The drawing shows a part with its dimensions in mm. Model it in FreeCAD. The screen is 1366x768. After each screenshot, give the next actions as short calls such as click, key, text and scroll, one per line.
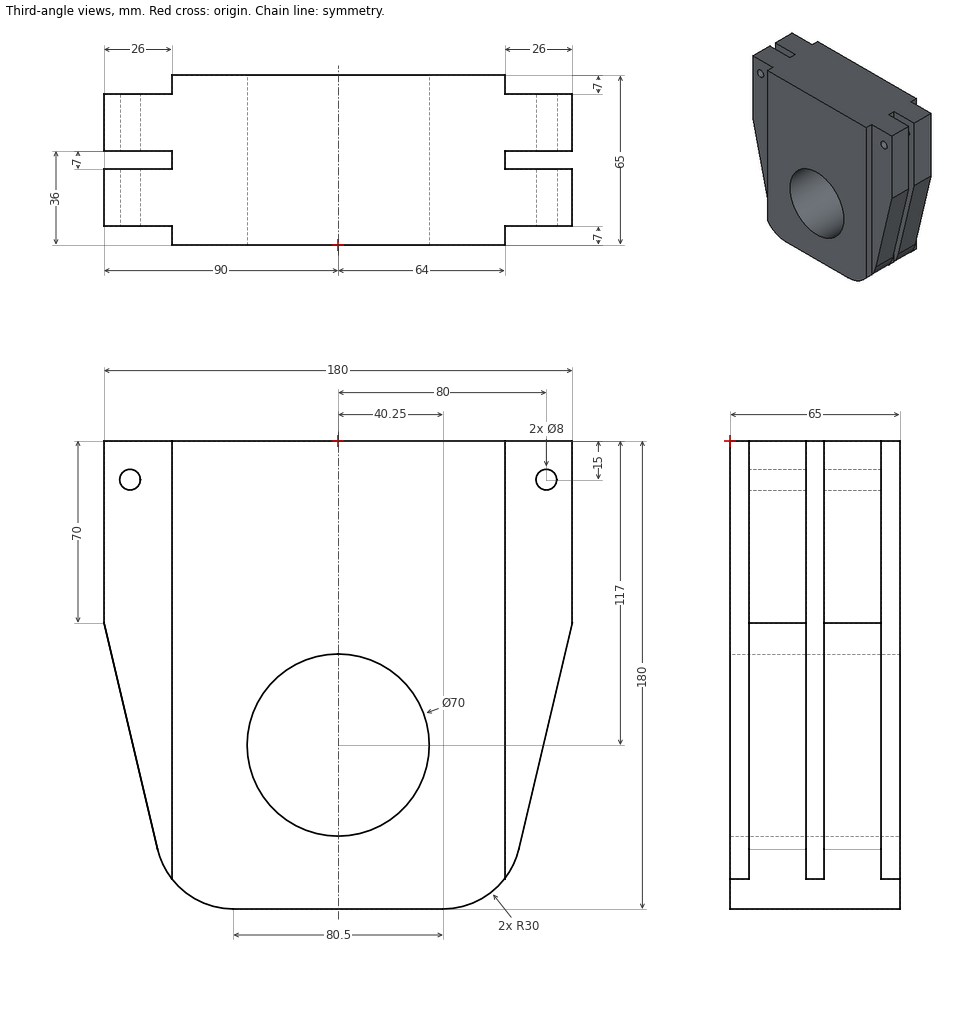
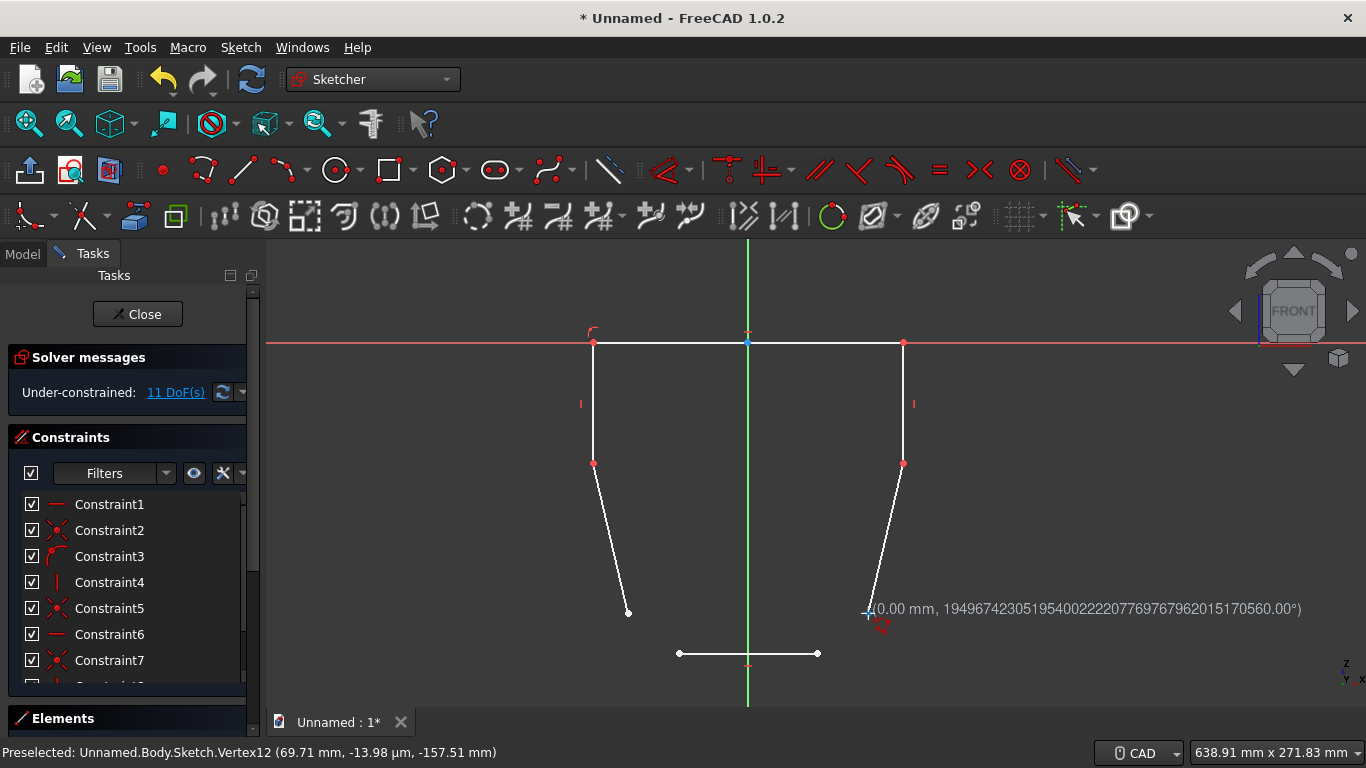
click(284, 170)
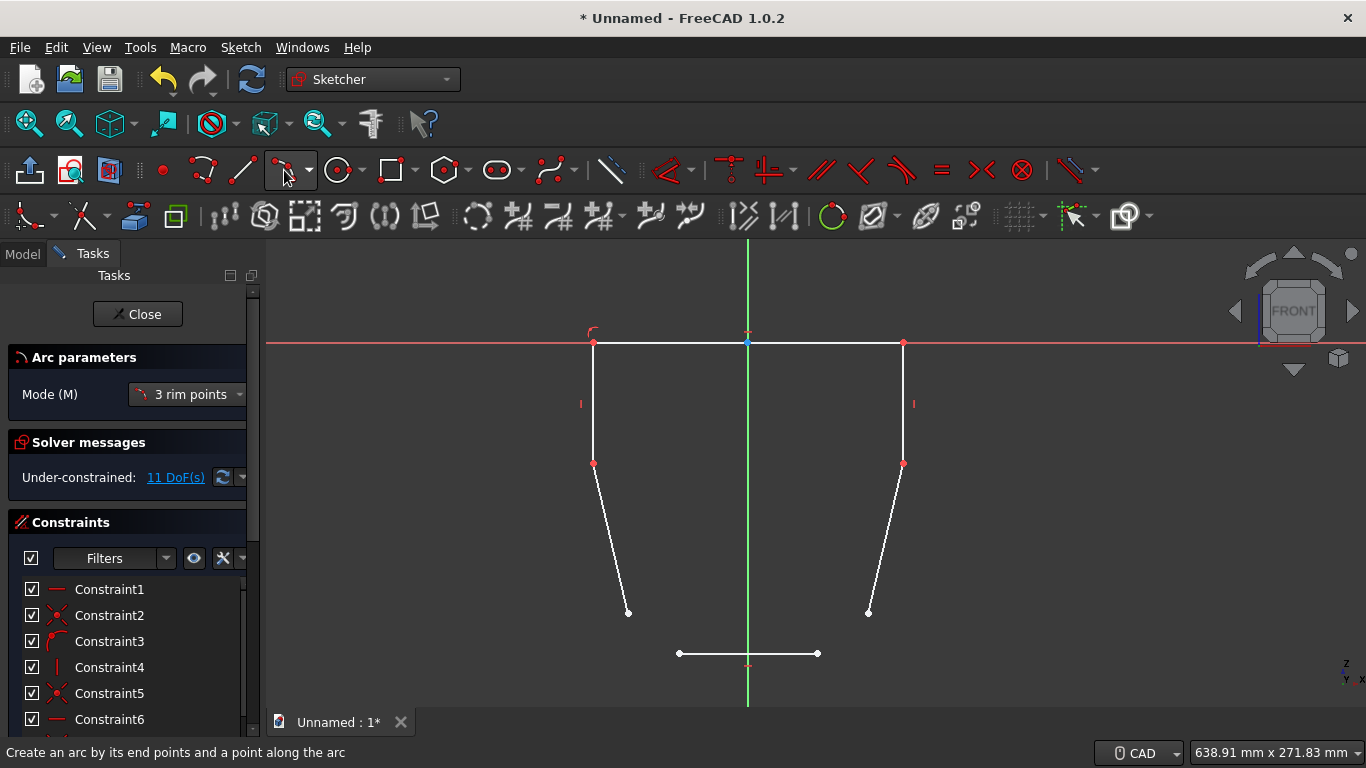
click(679, 654)
click(628, 614)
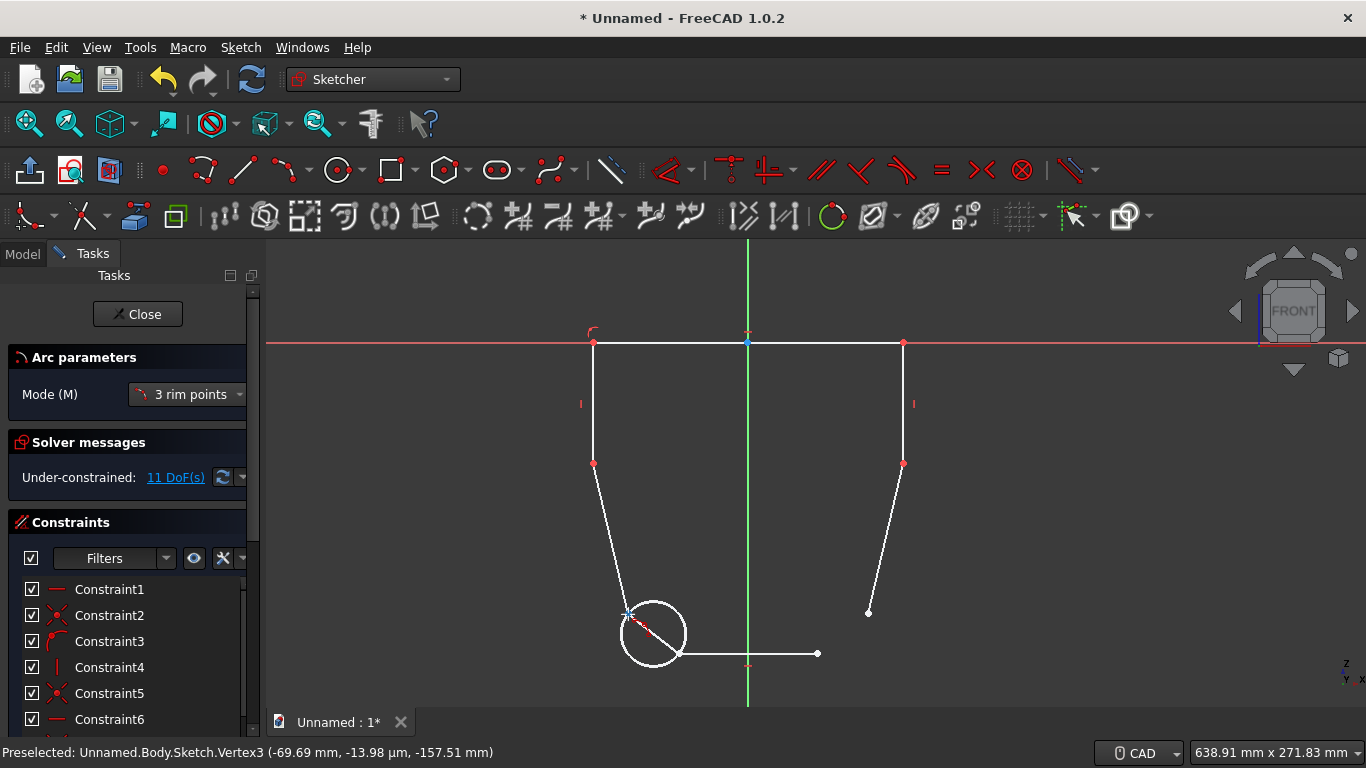
scroll(647, 642, up, 2)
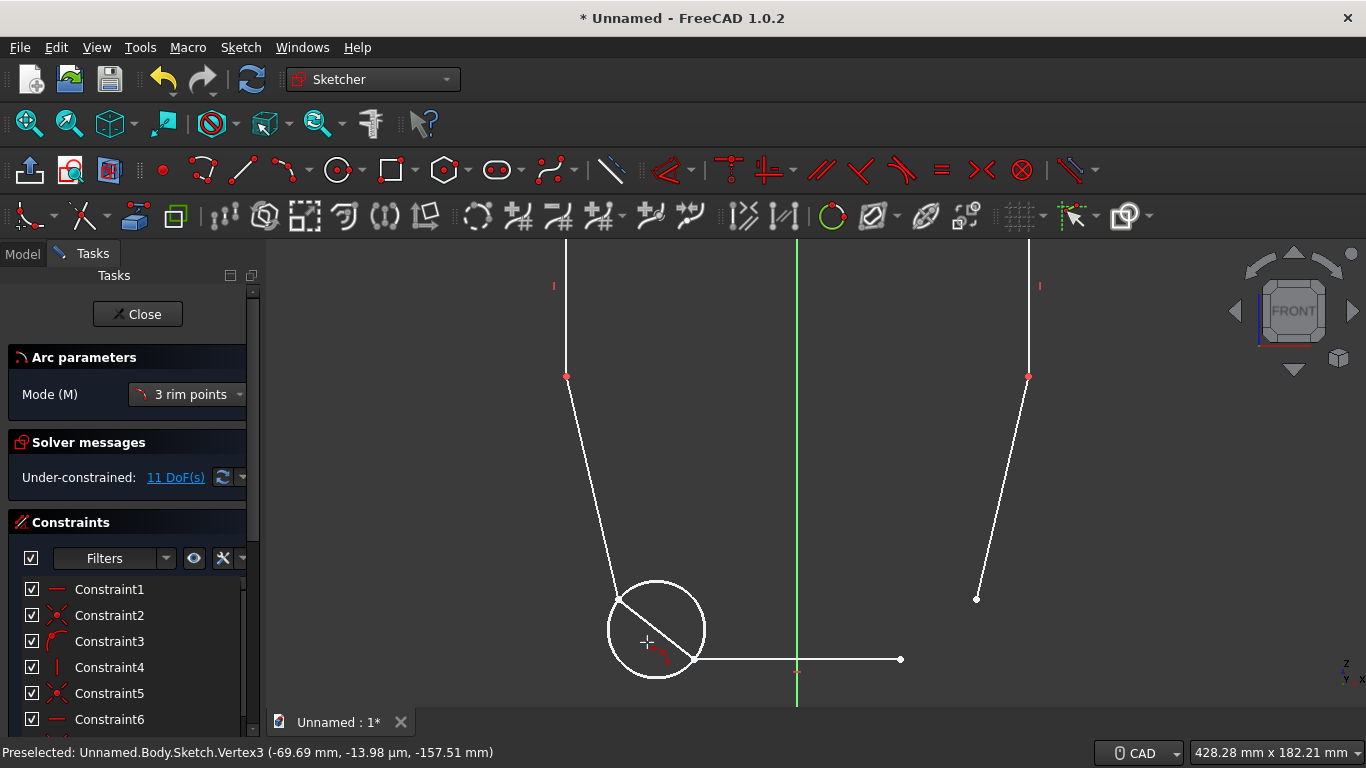
click(646, 641)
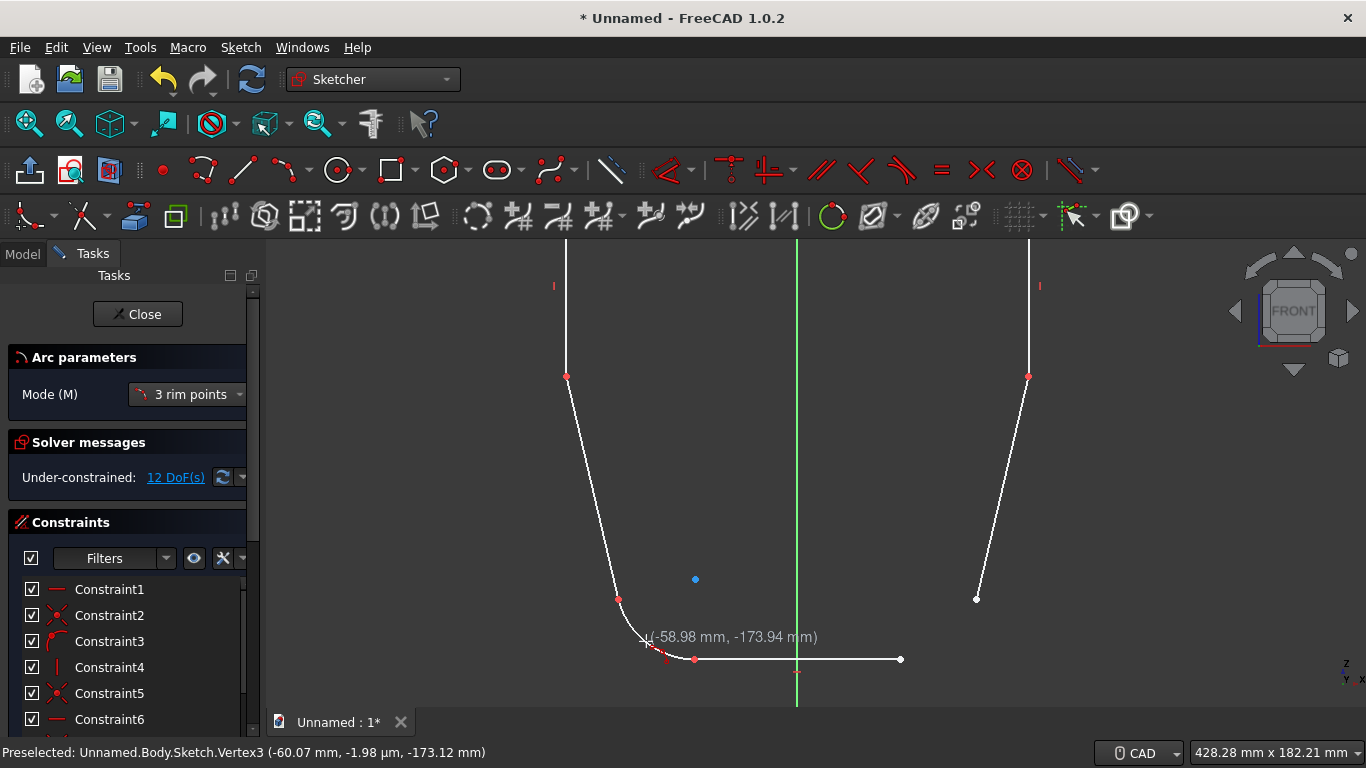
click(977, 600)
click(900, 659)
click(949, 641)
key(Escape)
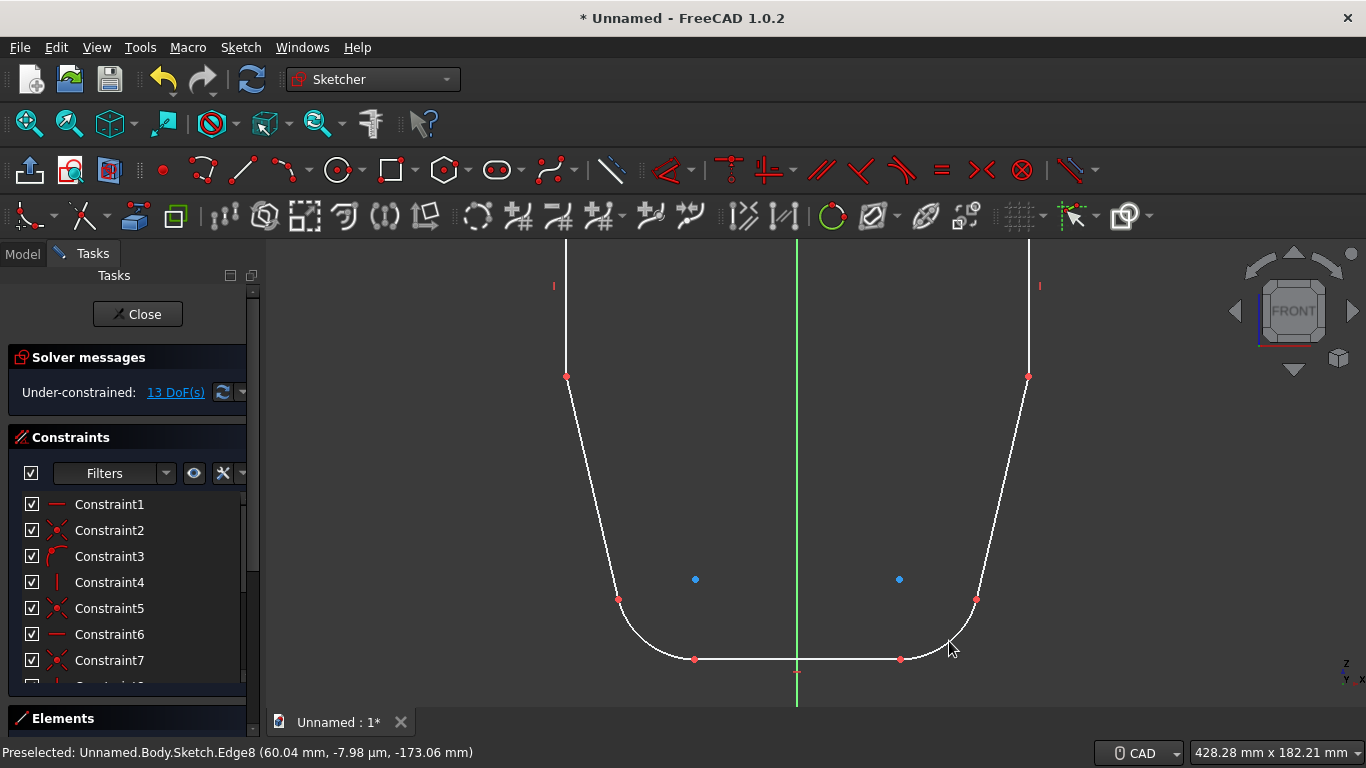
click(839, 659)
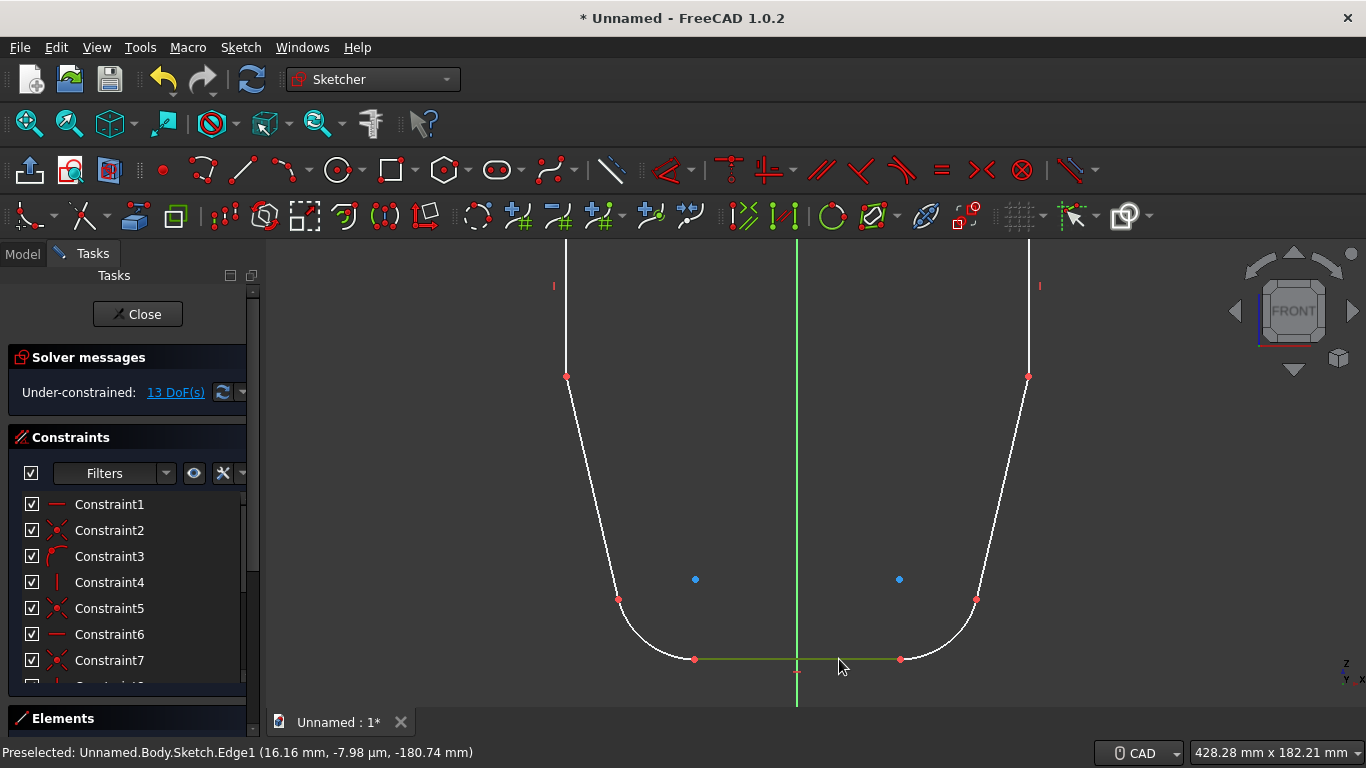
click(632, 628)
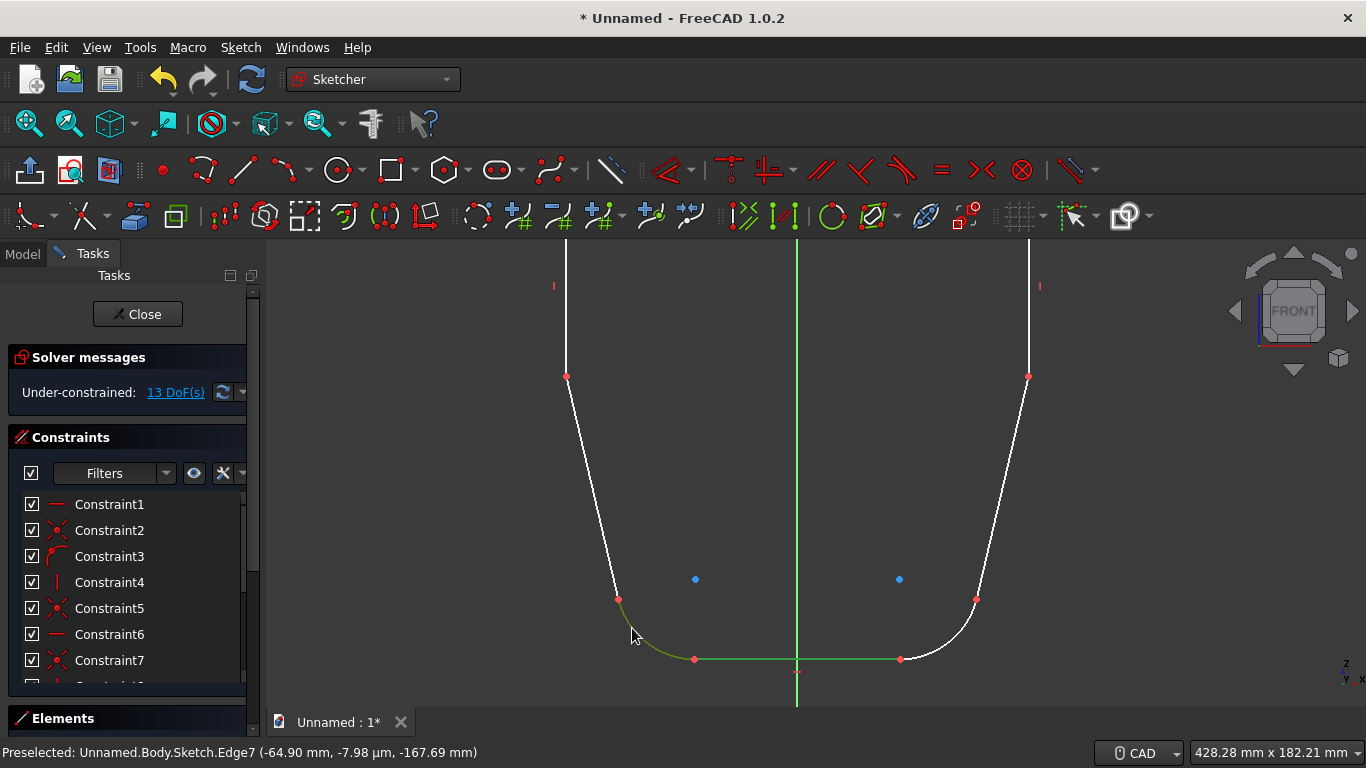
click(902, 170)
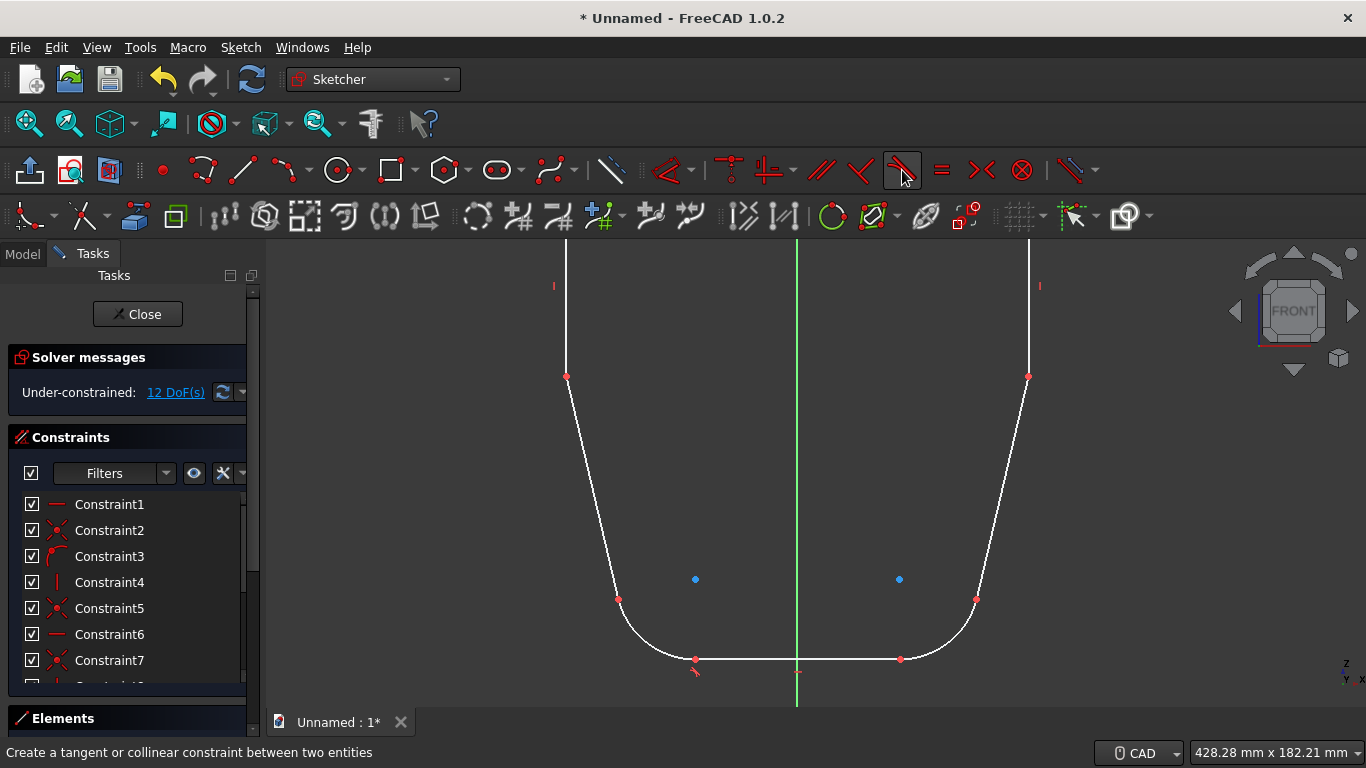
click(839, 659)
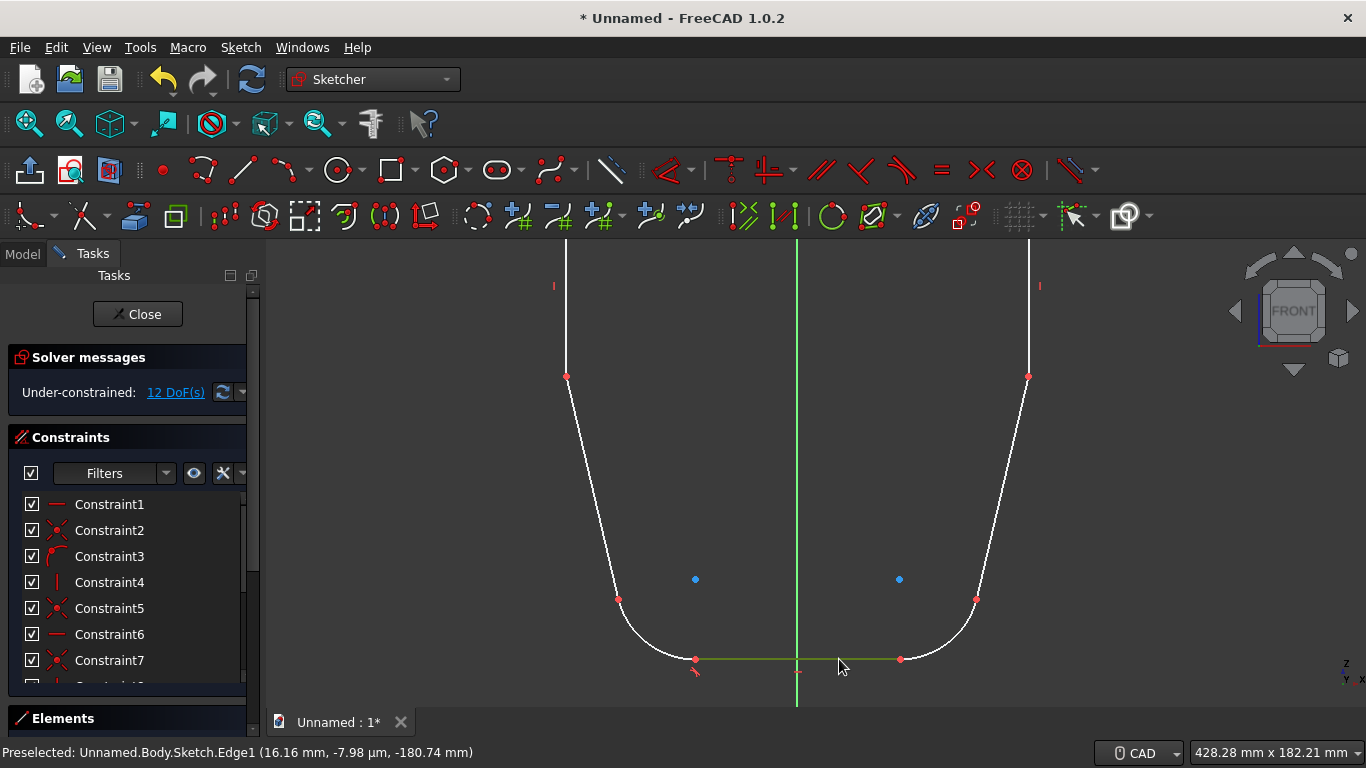
click(931, 653)